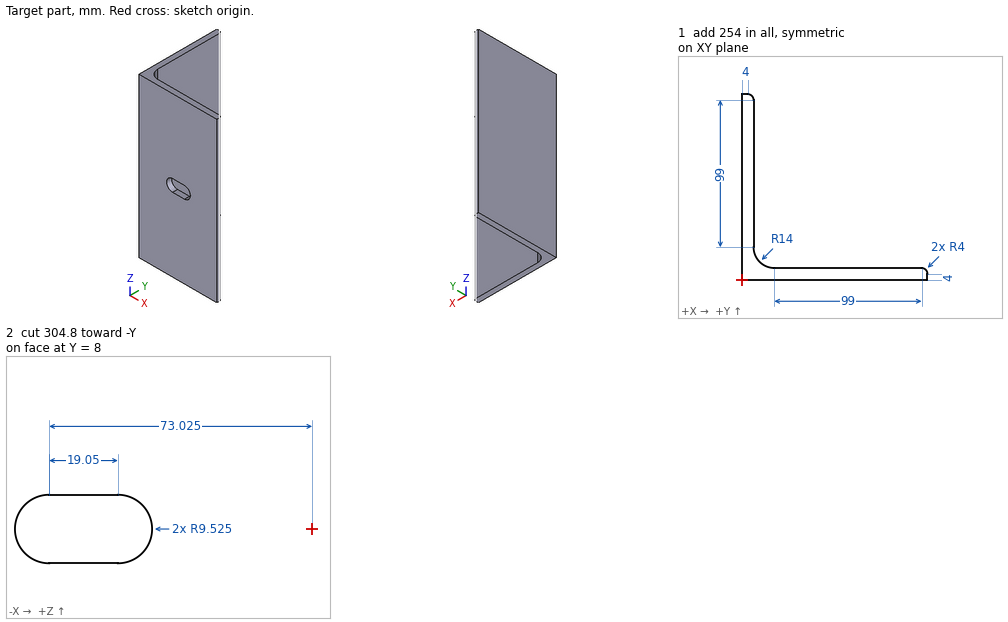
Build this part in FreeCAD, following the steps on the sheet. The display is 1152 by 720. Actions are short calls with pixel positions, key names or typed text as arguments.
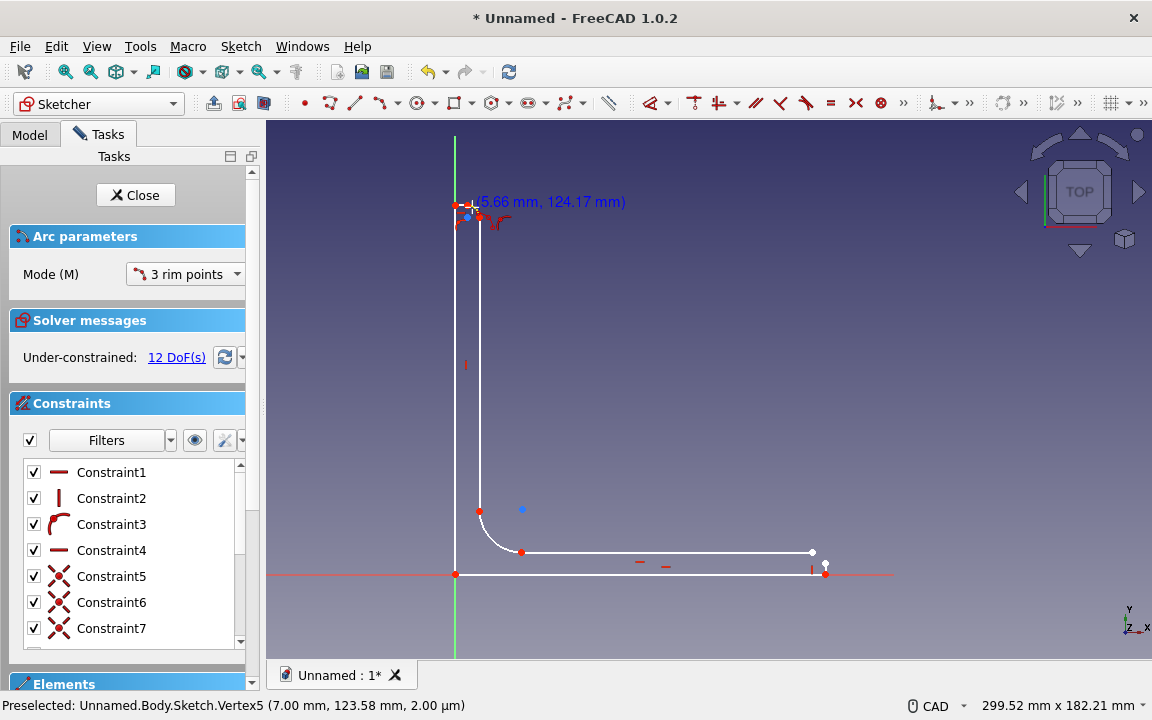
scroll(825, 563, up, 5)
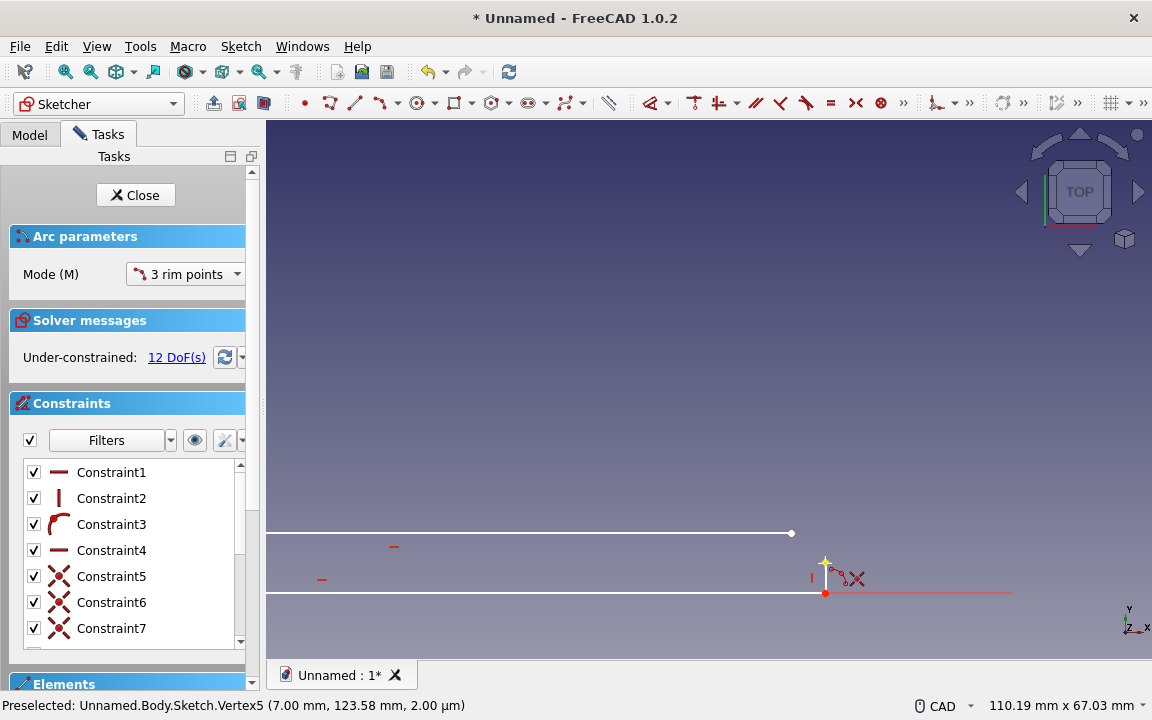
click(826, 563)
click(791, 533)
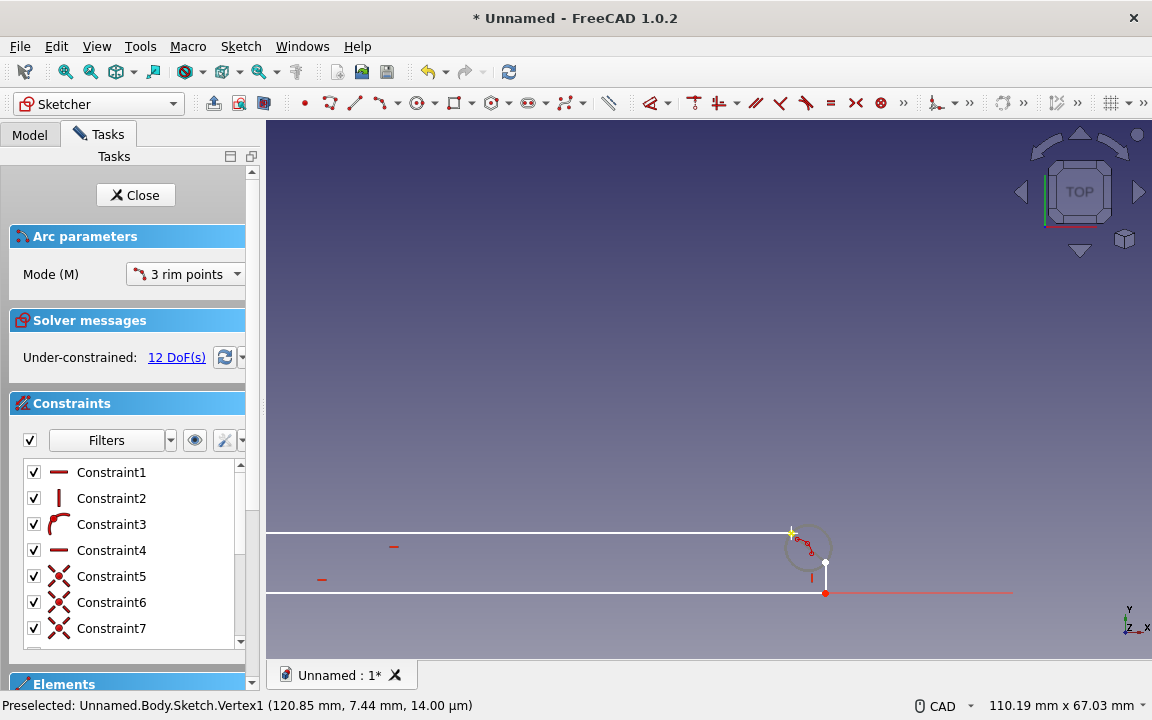
scroll(815, 538, up, 3)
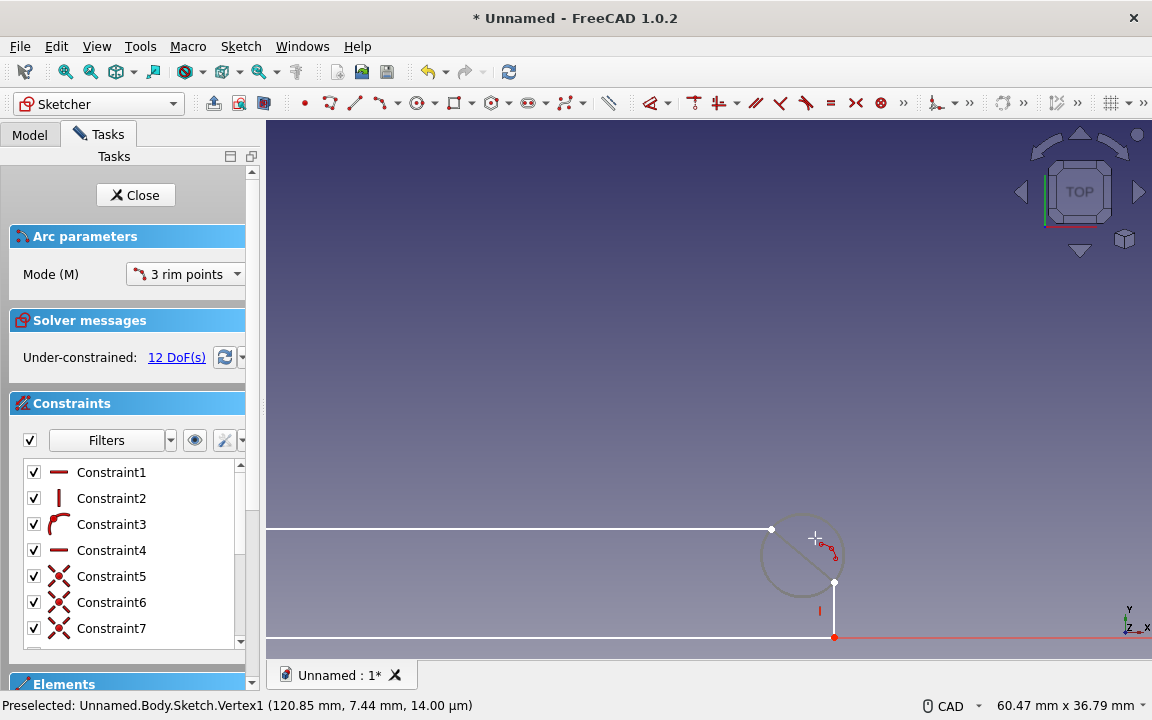
click(815, 538)
key(Escape)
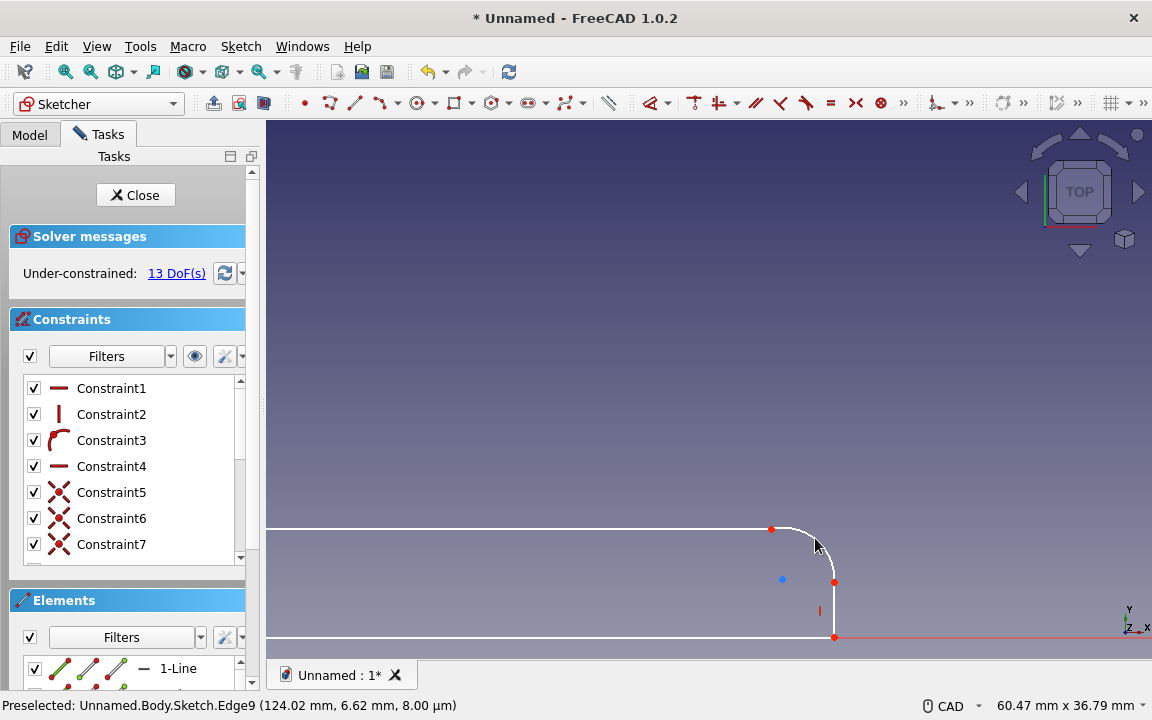
scroll(824, 558, down, 8)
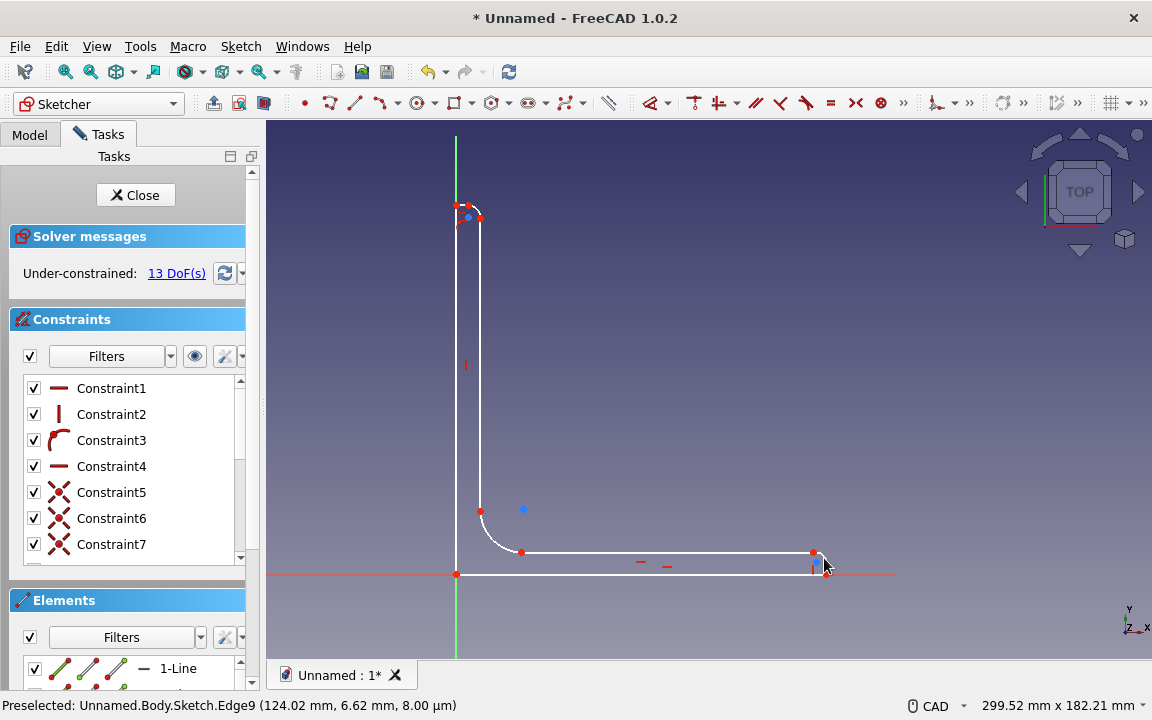
click(726, 553)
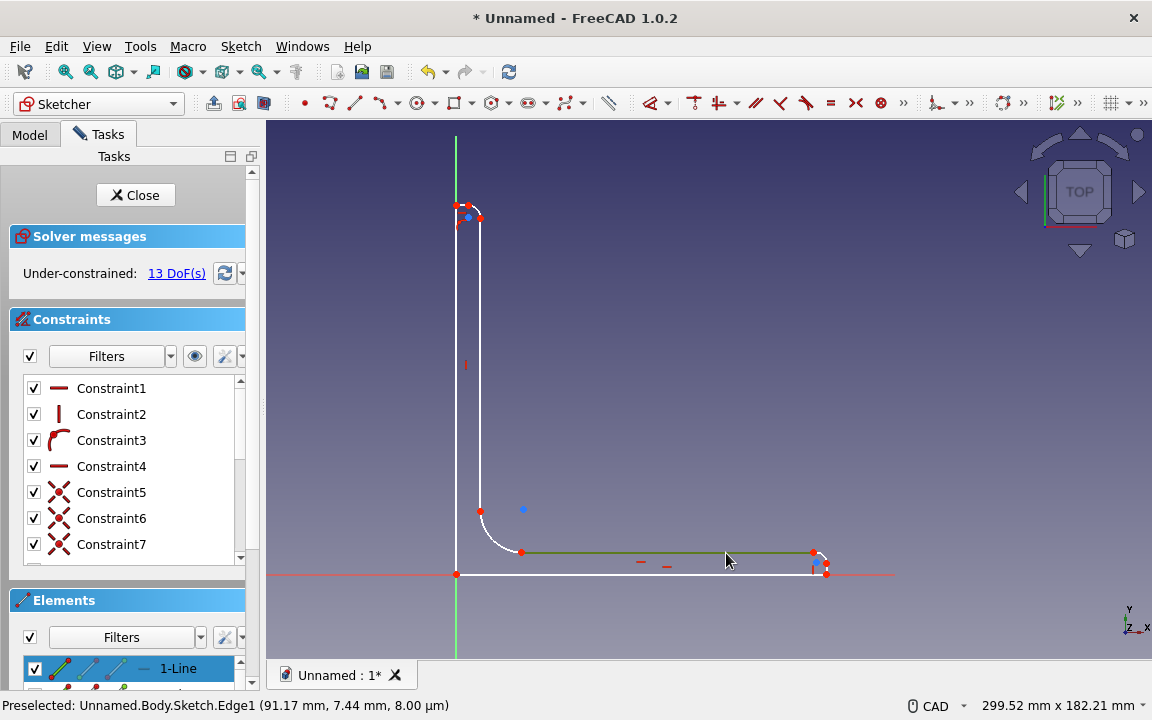
click(485, 530)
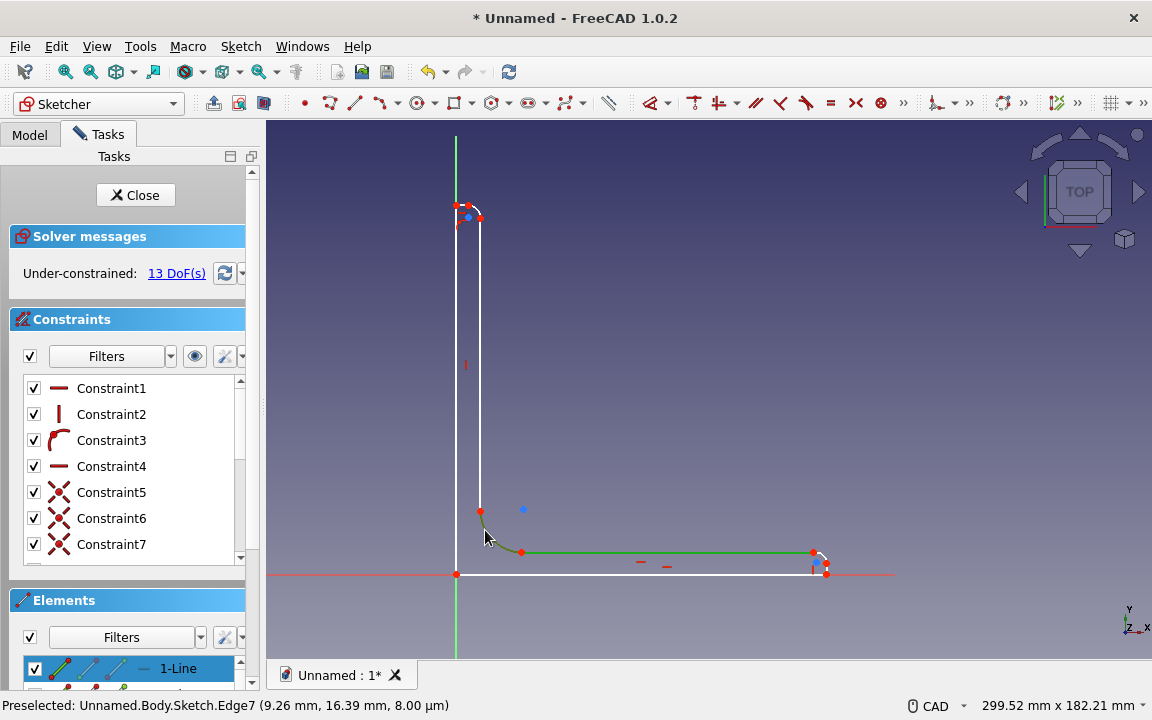
click(806, 104)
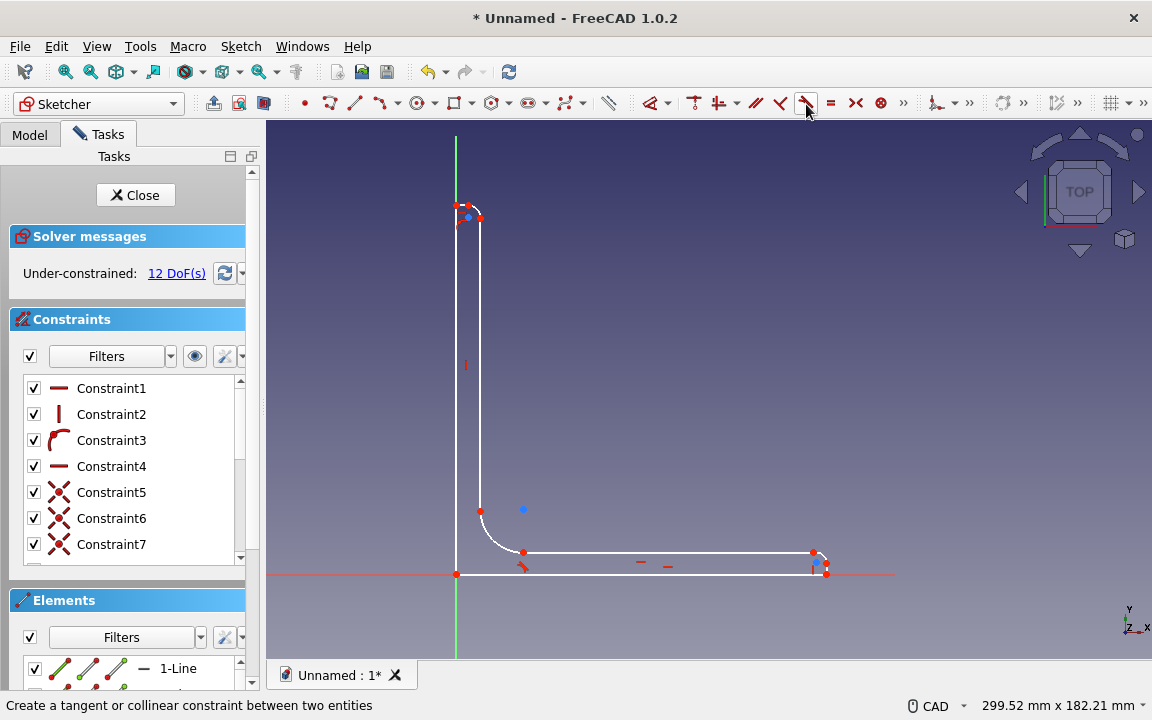
click(727, 553)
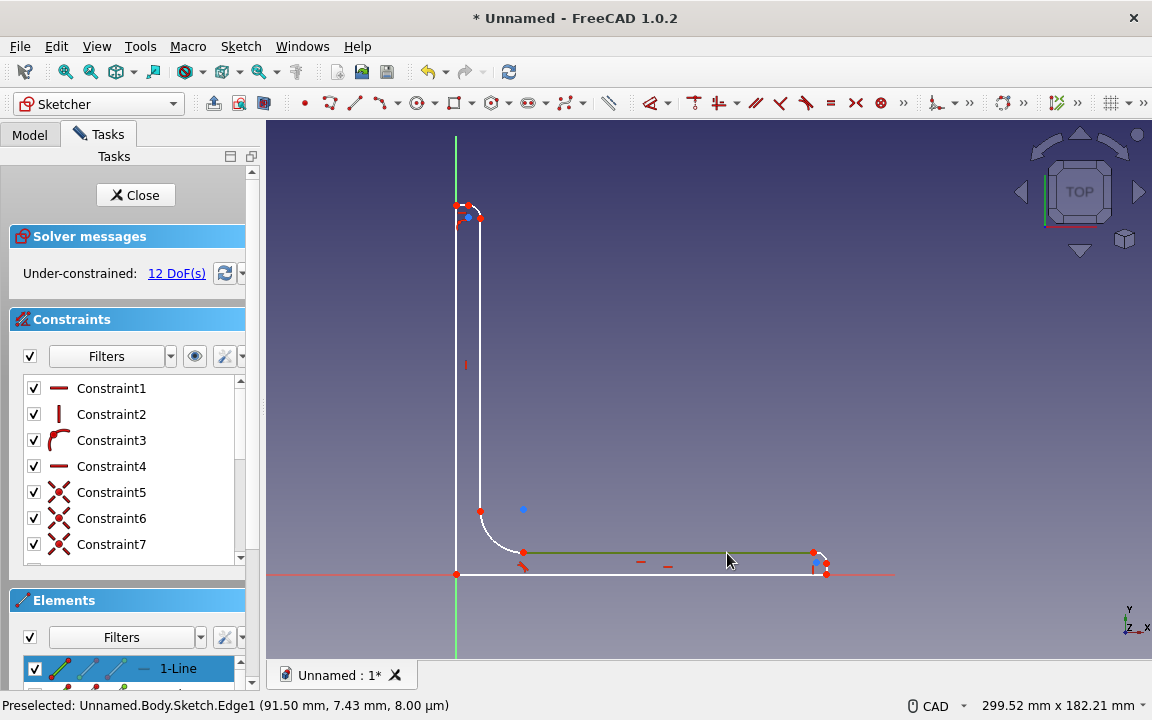
scroll(823, 555, up, 2)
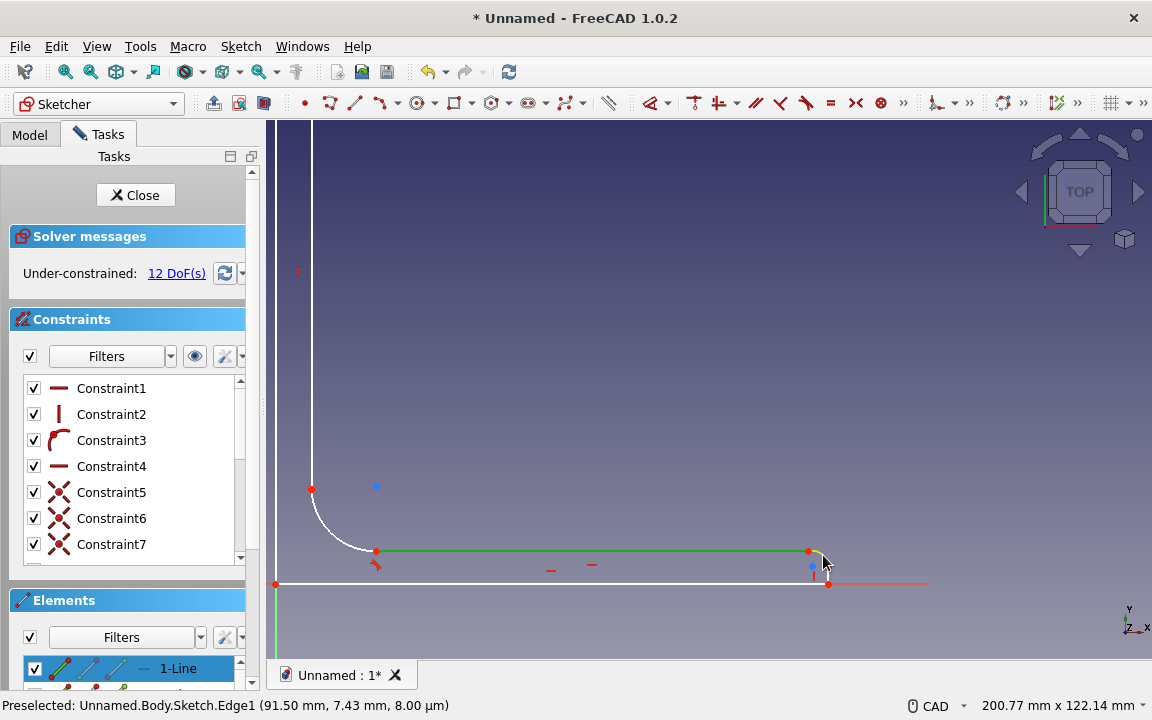
click(823, 555)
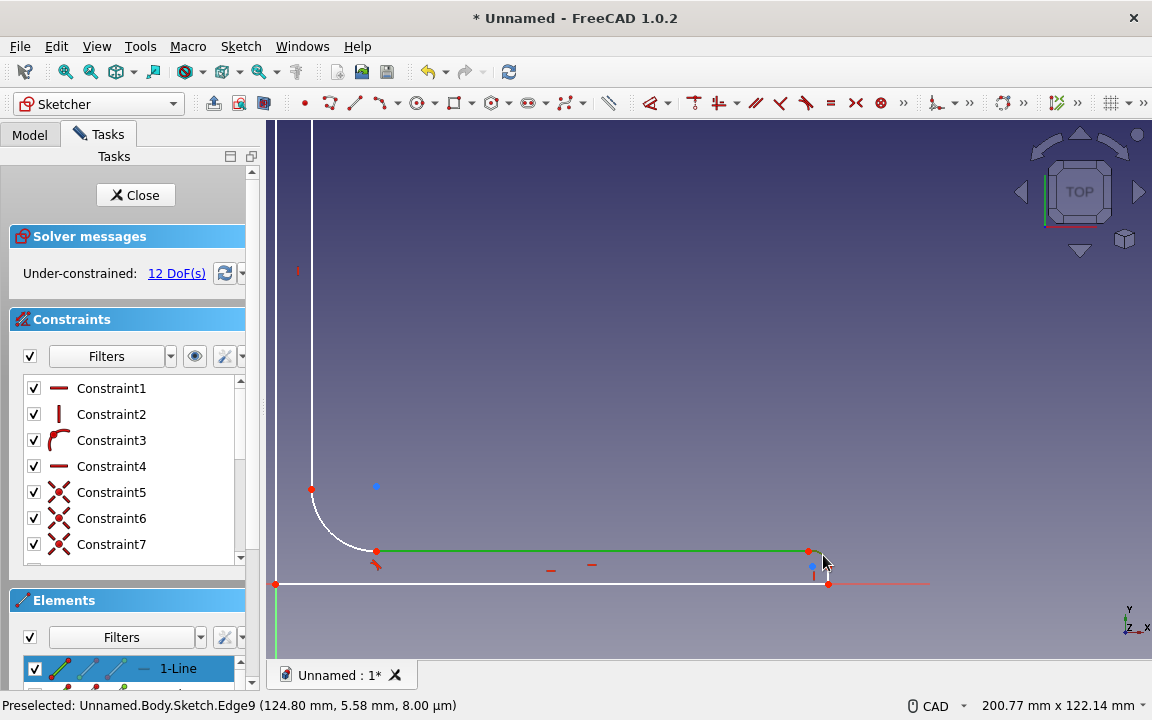
click(806, 104)